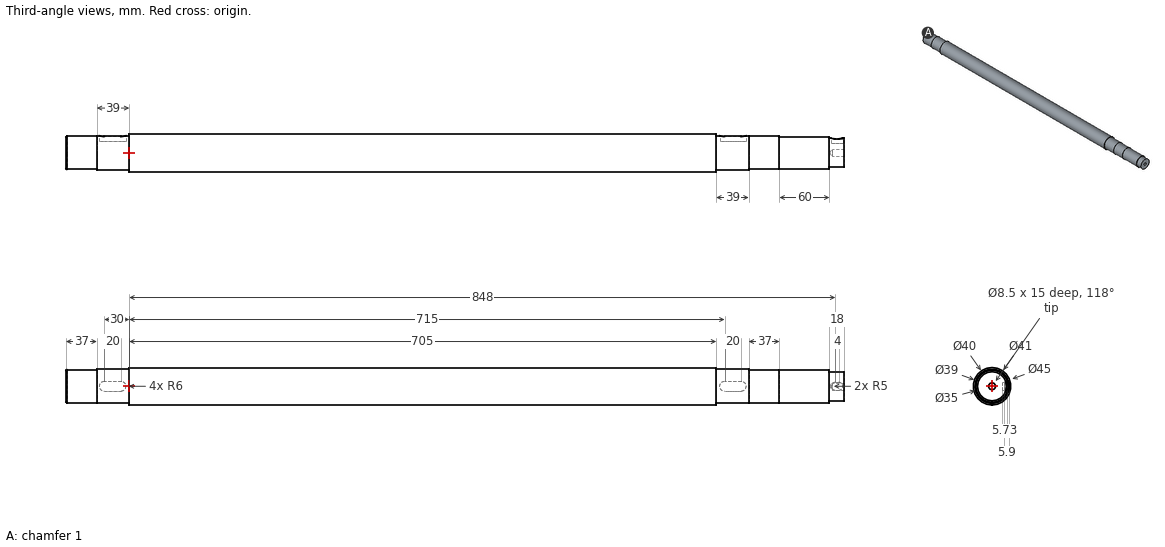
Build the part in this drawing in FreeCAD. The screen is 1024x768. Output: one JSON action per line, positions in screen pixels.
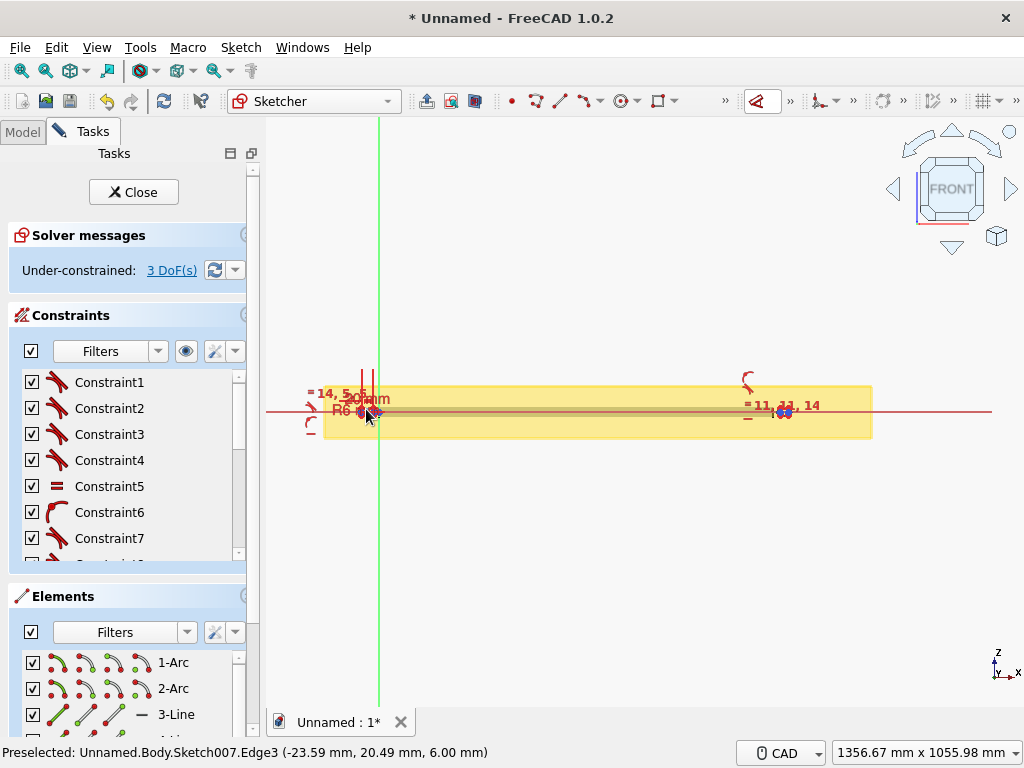
{"action": "scroll", "coordinate": [783, 409], "scroll_direction": "up", "scroll_amount": 10}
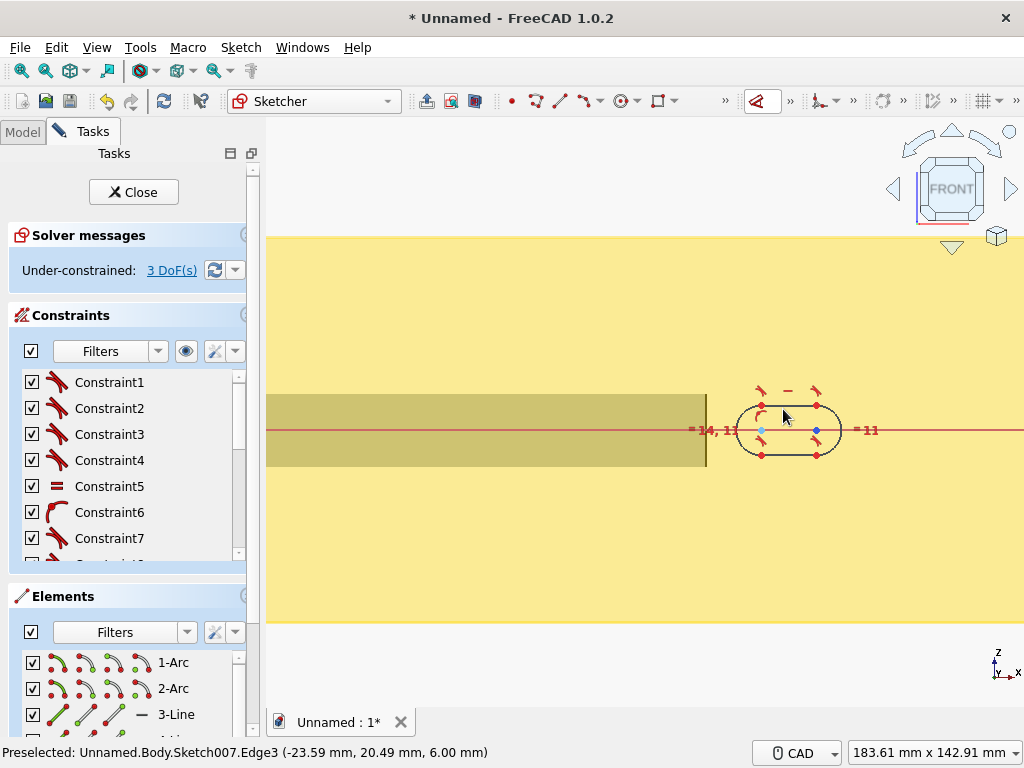
{"action": "left_click", "coordinate": [778, 406]}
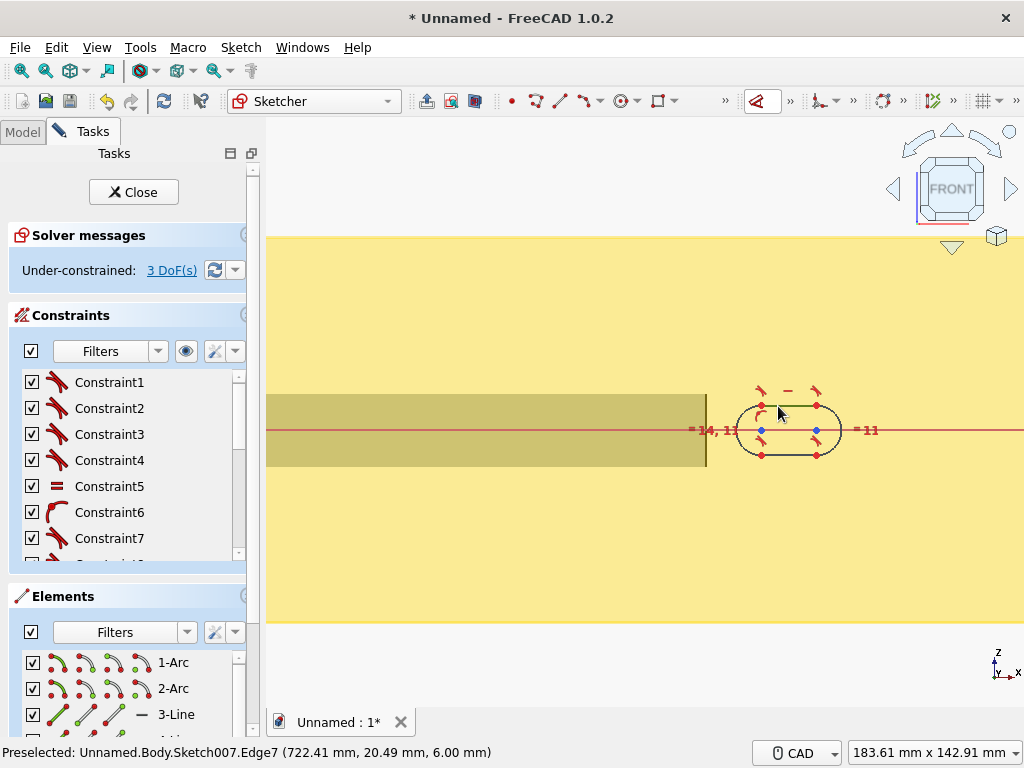
{"action": "key", "text": "l"}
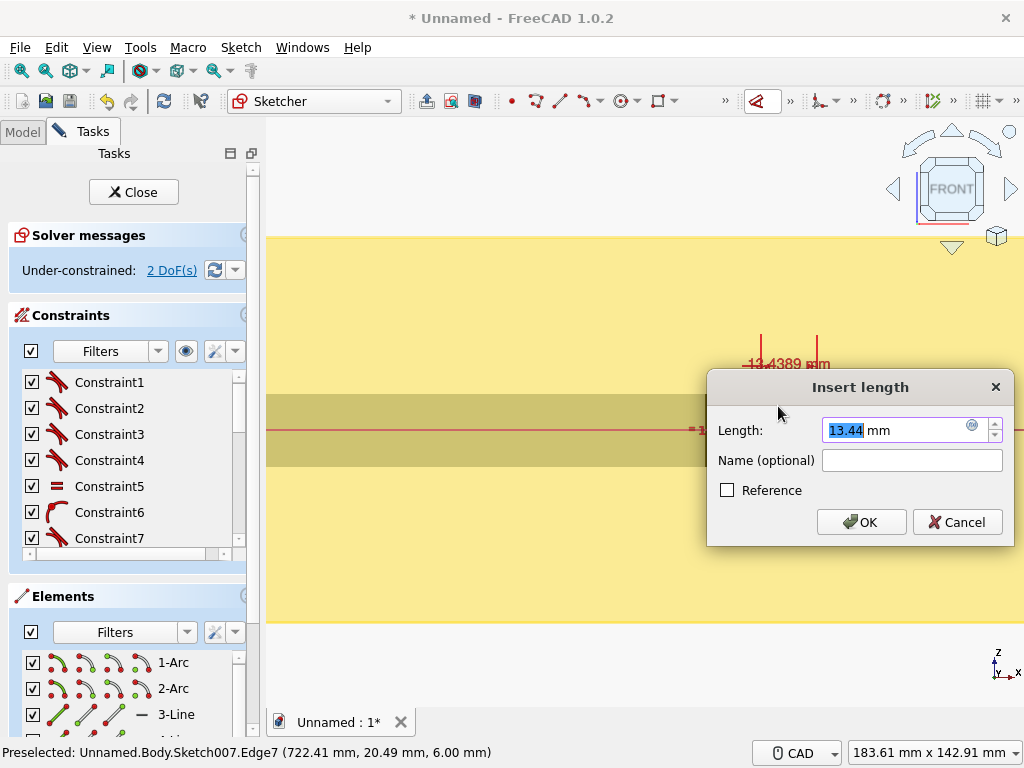
{"action": "type", "text": "20"}
{"action": "key", "text": "Return"}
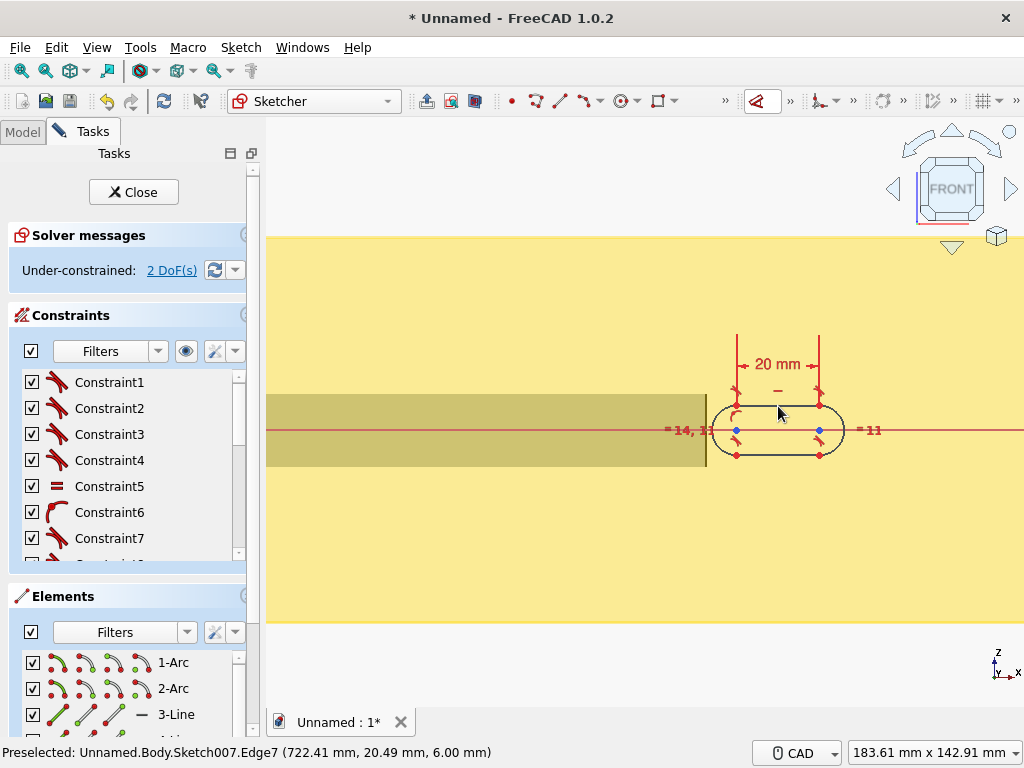
{"action": "scroll", "coordinate": [784, 409], "scroll_direction": "down", "scroll_amount": 10}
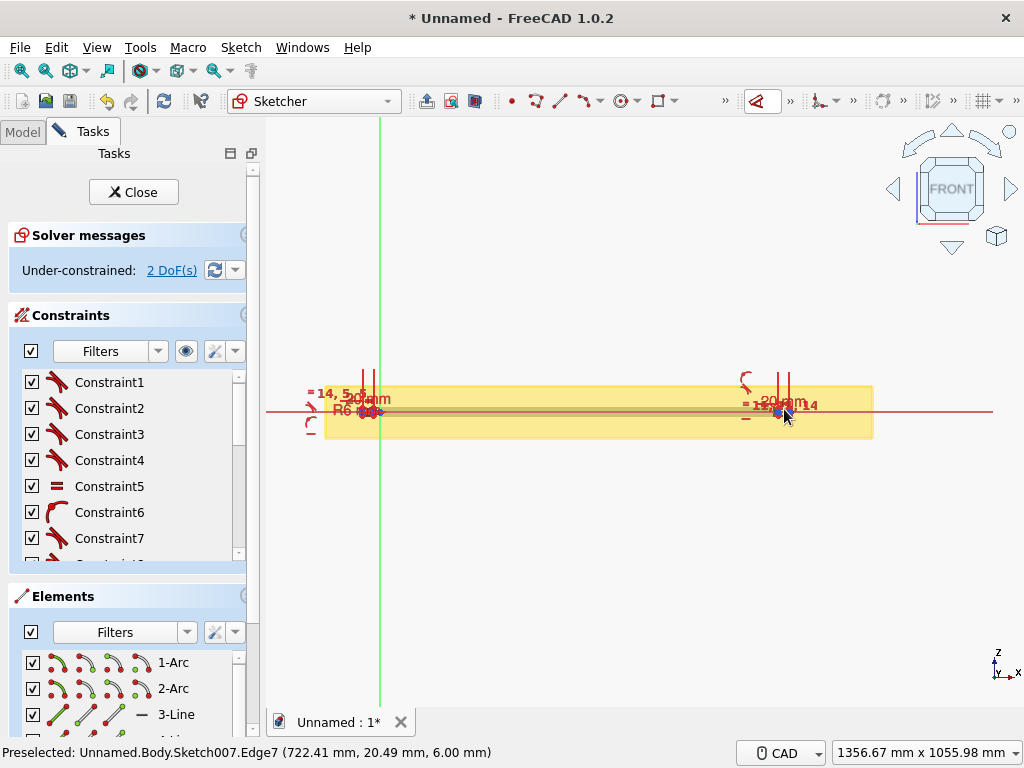
{"action": "scroll", "coordinate": [363, 409], "scroll_direction": "up", "scroll_amount": 7}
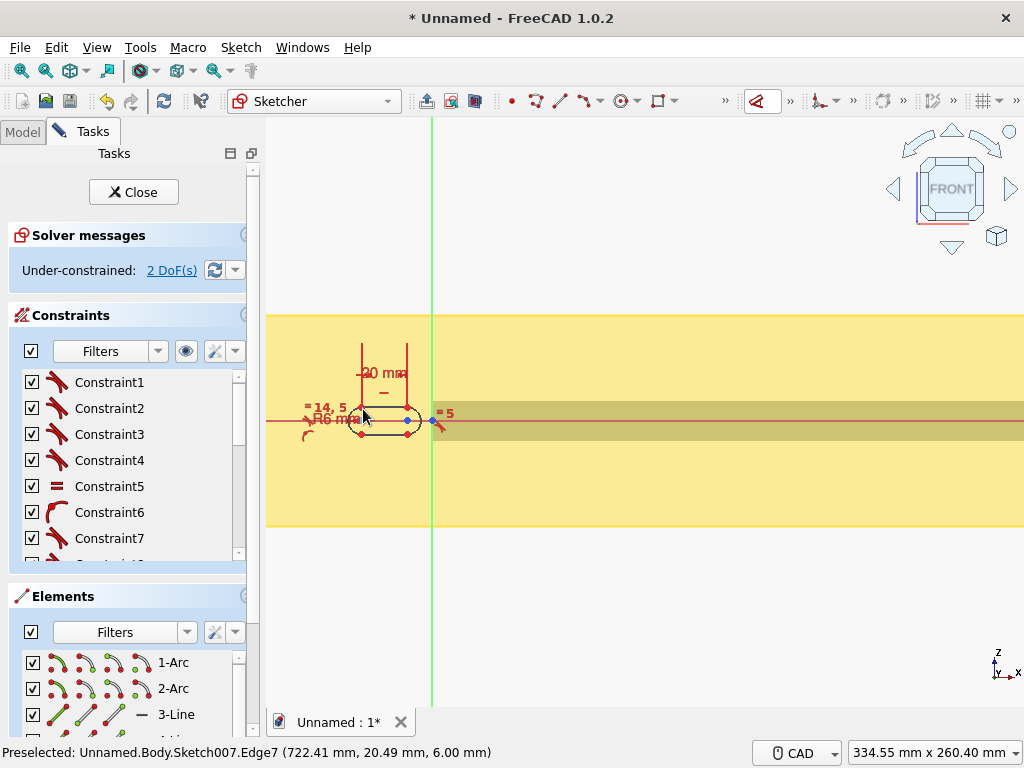
{"action": "left_click", "coordinate": [362, 407]}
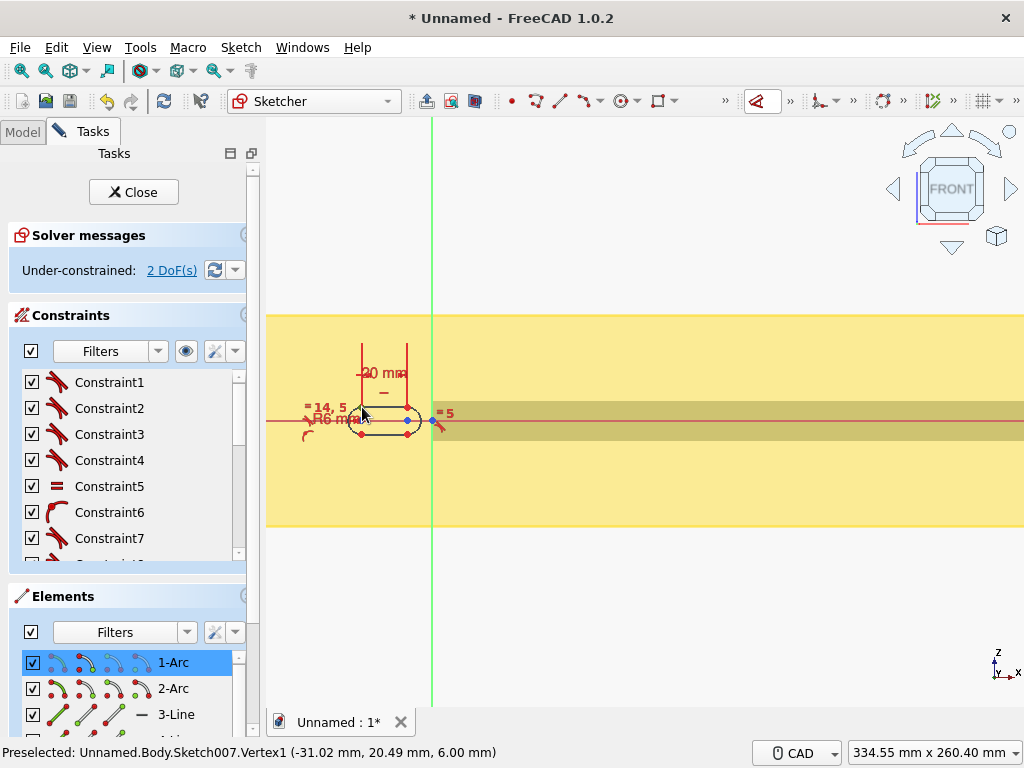
{"action": "key", "text": "l"}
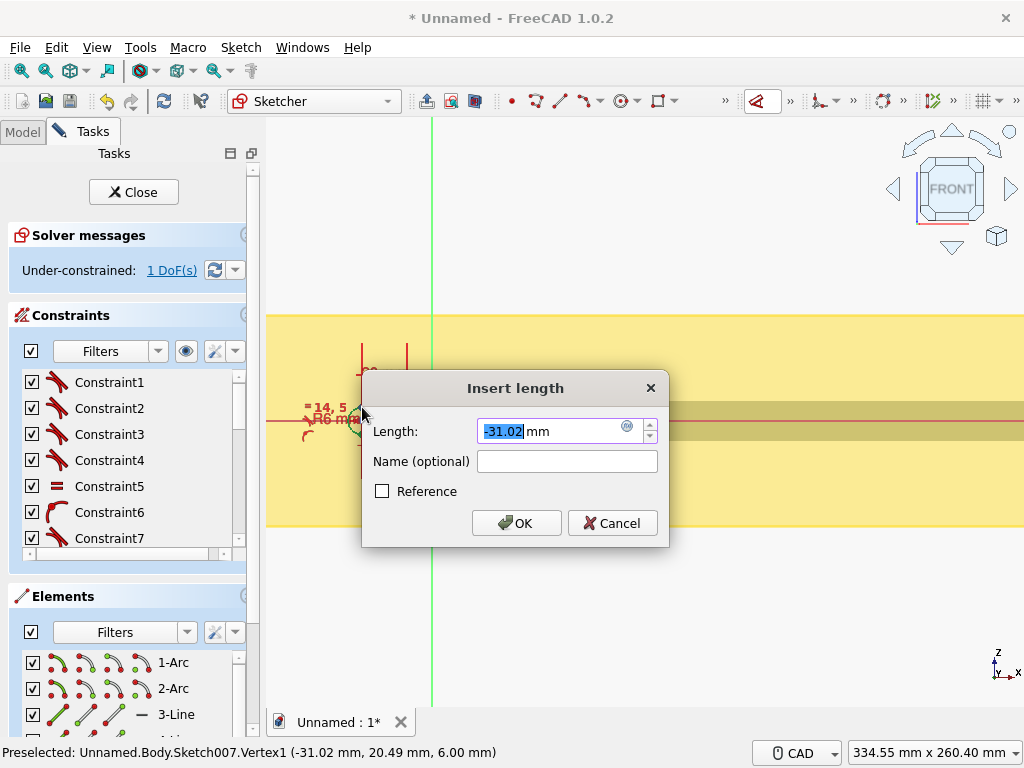
{"action": "type", "text": "-30"}
{"action": "key", "text": "Return"}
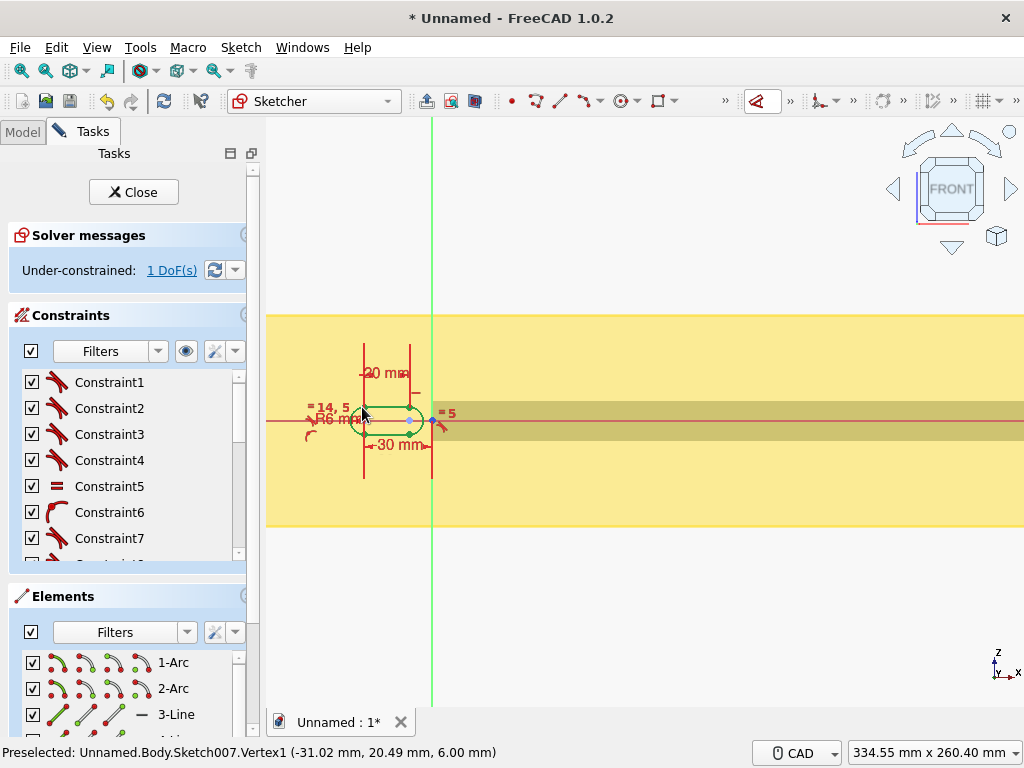
{"action": "scroll", "coordinate": [362, 409], "scroll_direction": "down", "scroll_amount": 7}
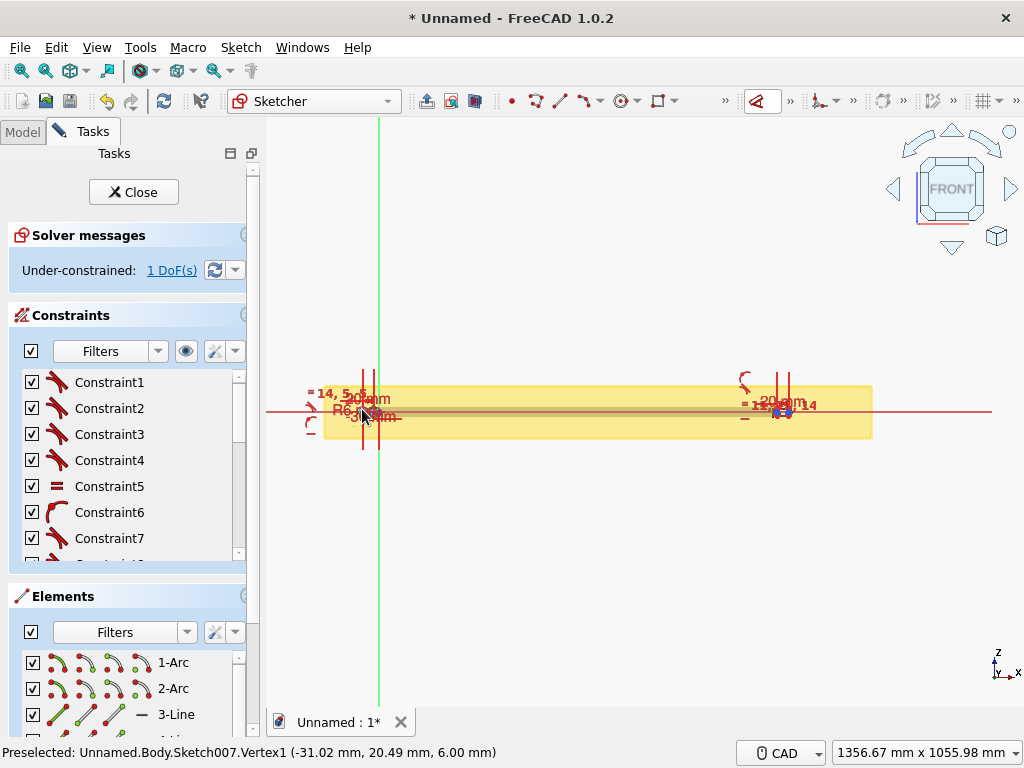
{"action": "scroll", "coordinate": [777, 409], "scroll_direction": "up", "scroll_amount": 7}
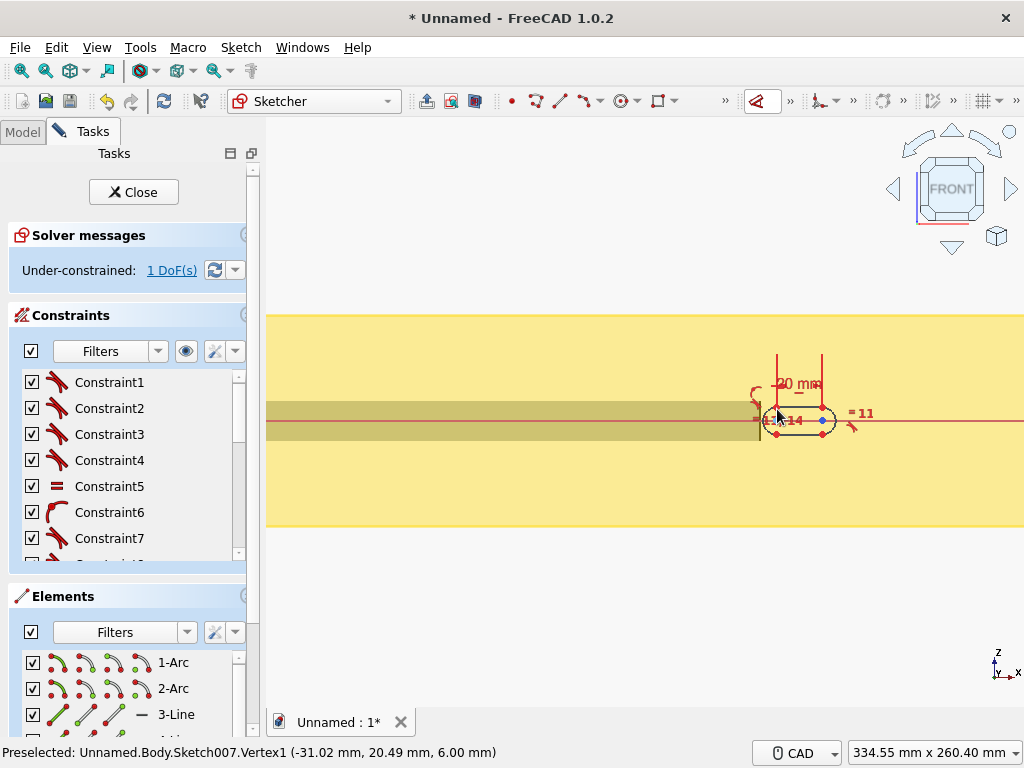
{"action": "left_click", "coordinate": [777, 407]}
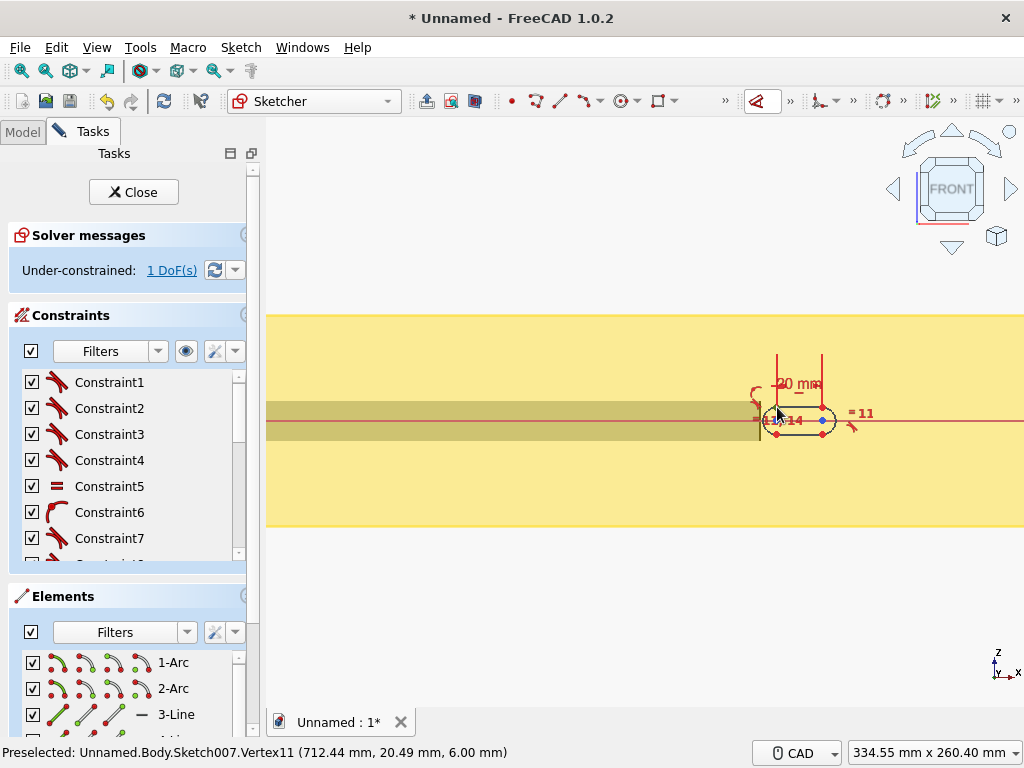
{"action": "left_click", "coordinate": [776, 102]}